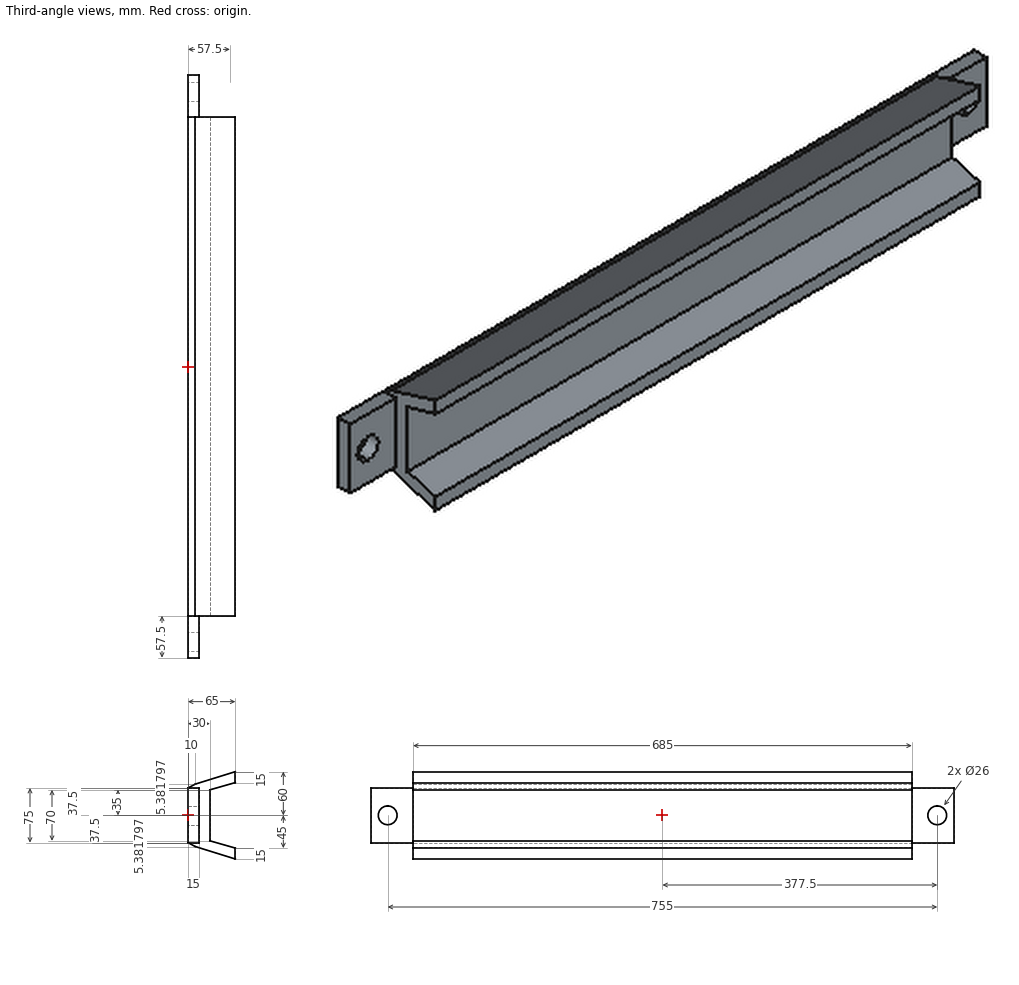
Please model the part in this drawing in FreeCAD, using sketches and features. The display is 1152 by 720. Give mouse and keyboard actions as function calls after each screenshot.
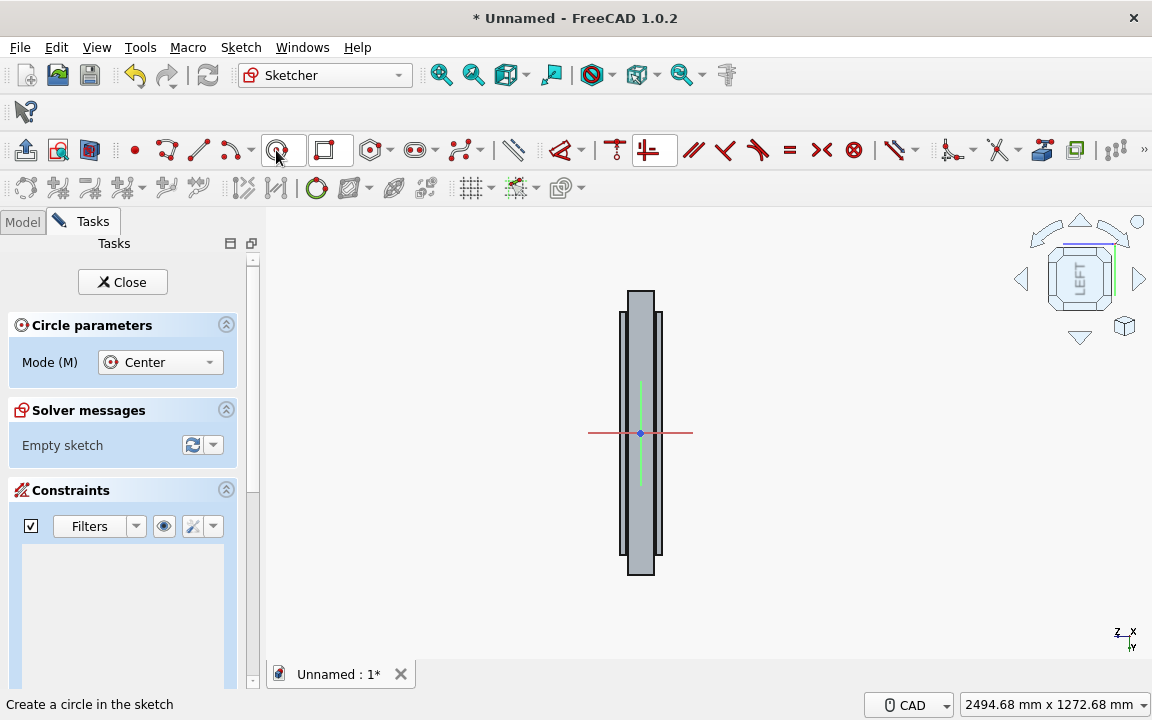
scroll(641, 567, up, 8)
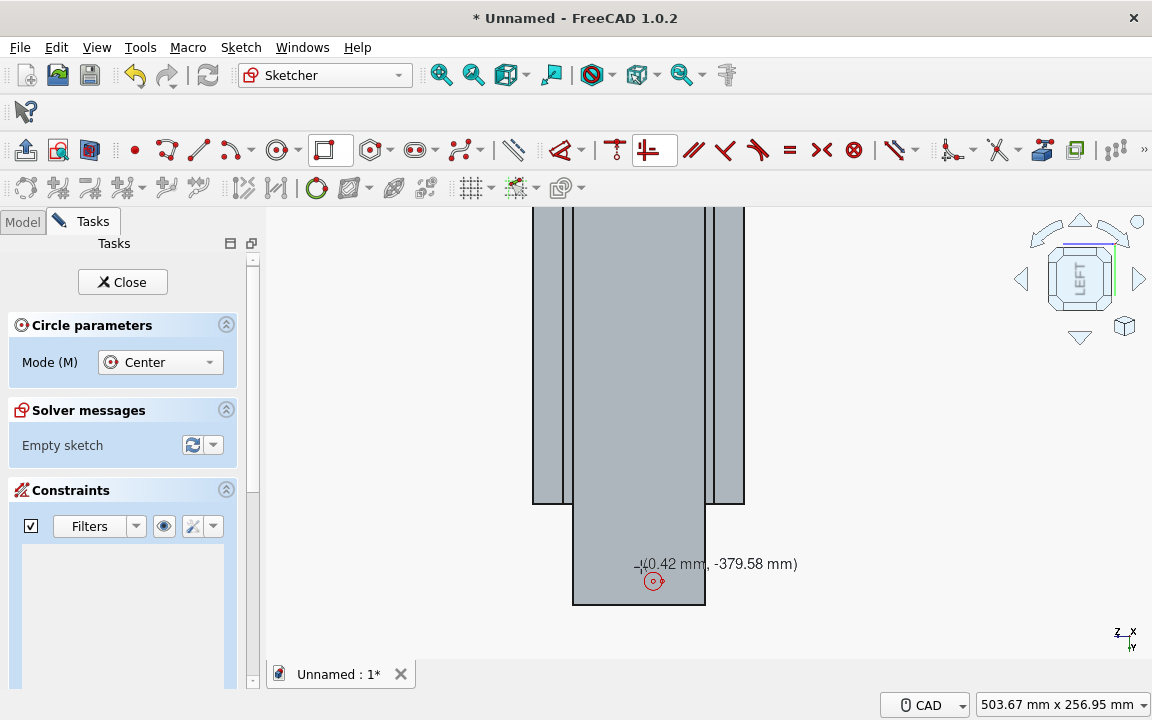
scroll(641, 568, down, 8)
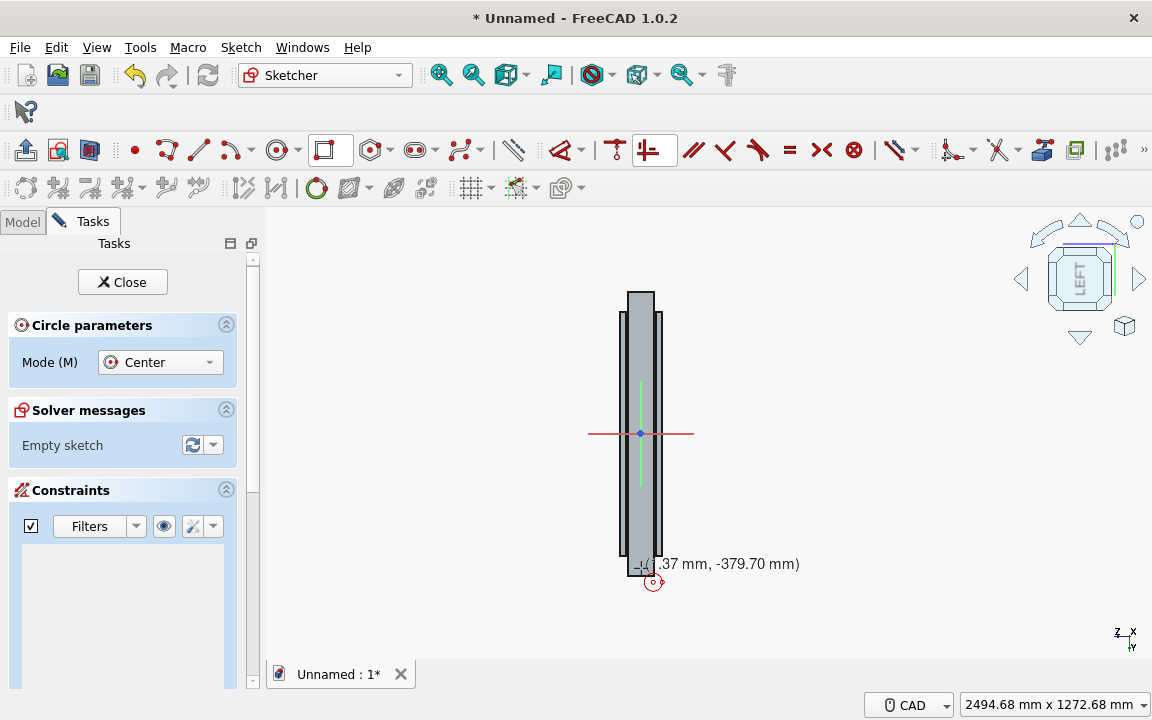
click(641, 568)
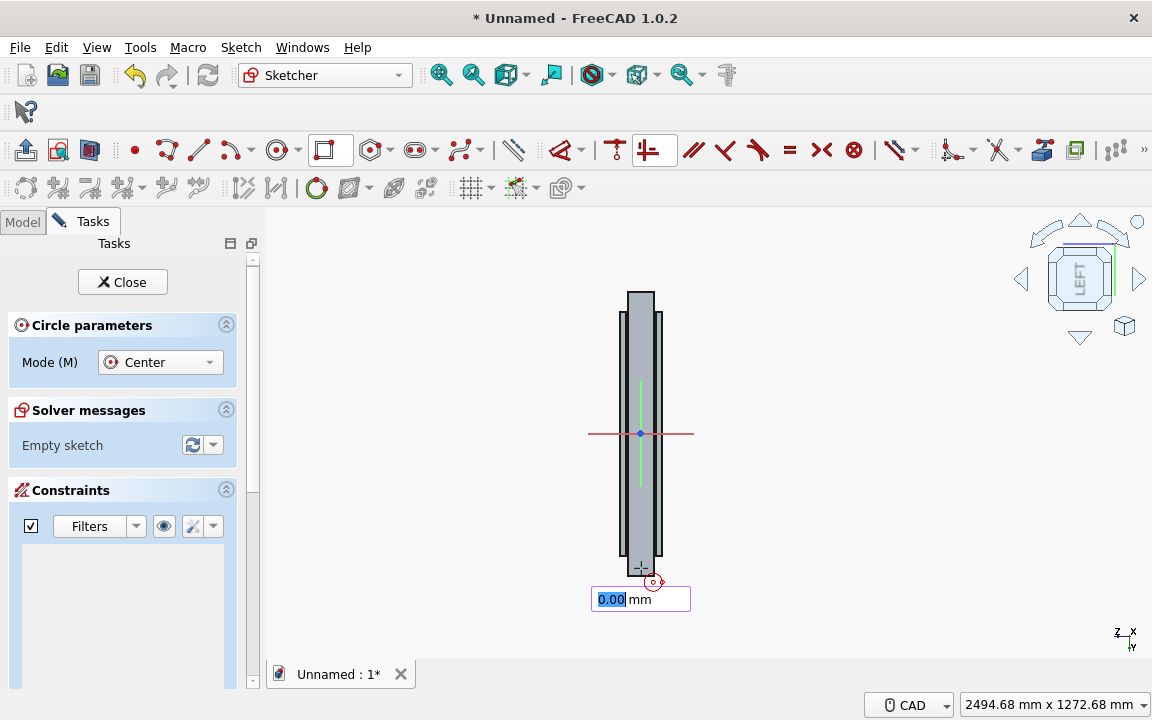
scroll(645, 566, up, 7)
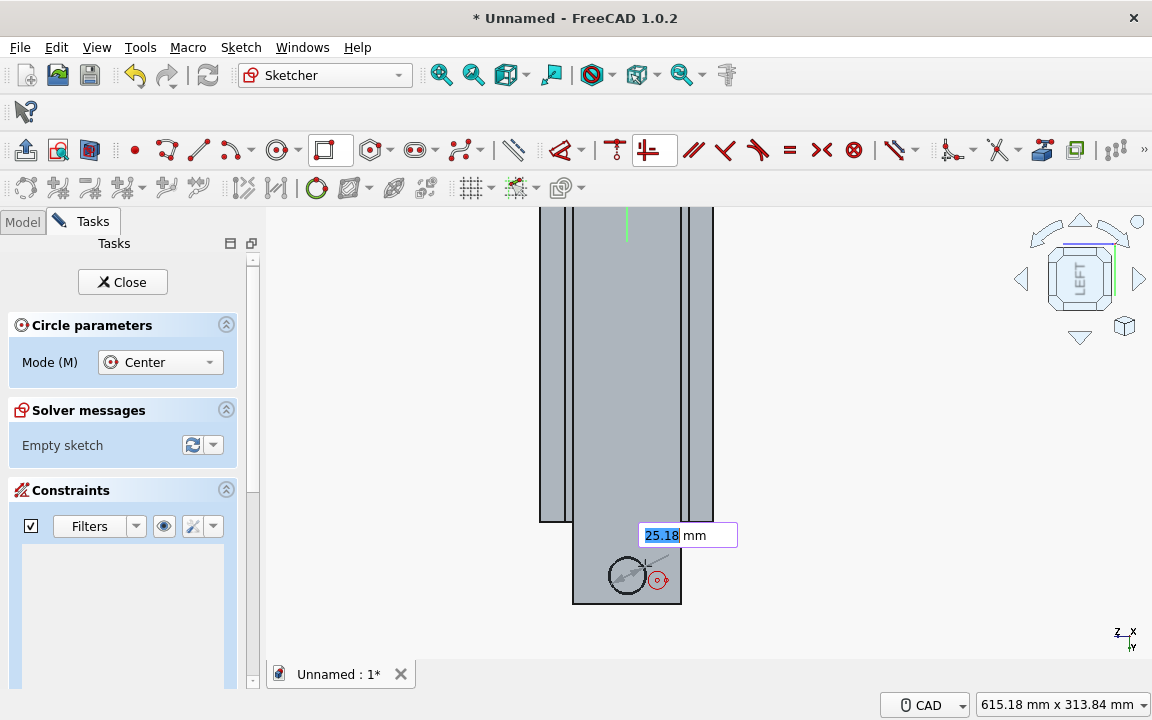
click(644, 566)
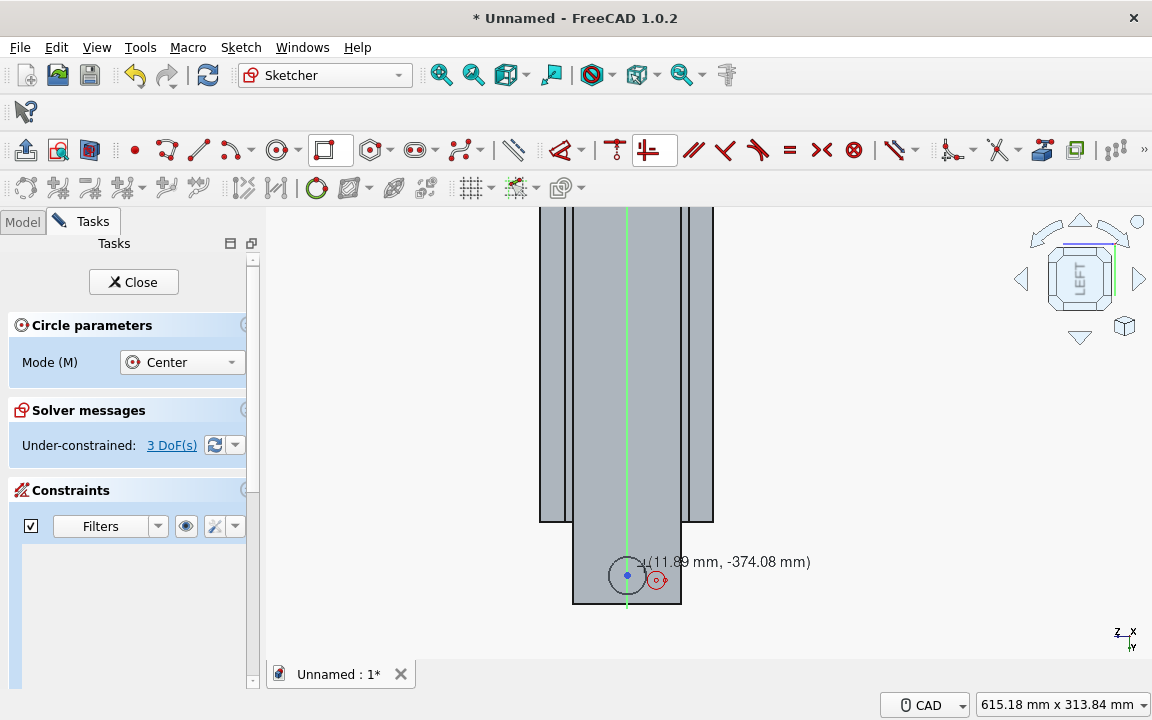
scroll(645, 565, down, 7)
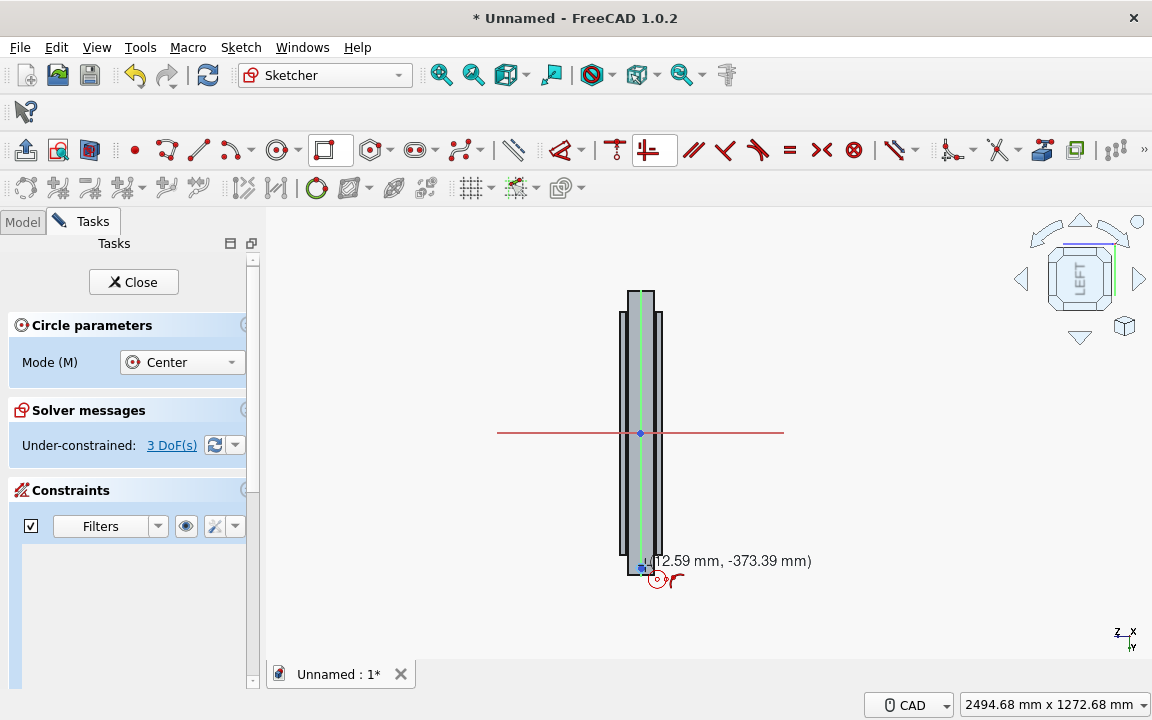
scroll(641, 299, up, 8)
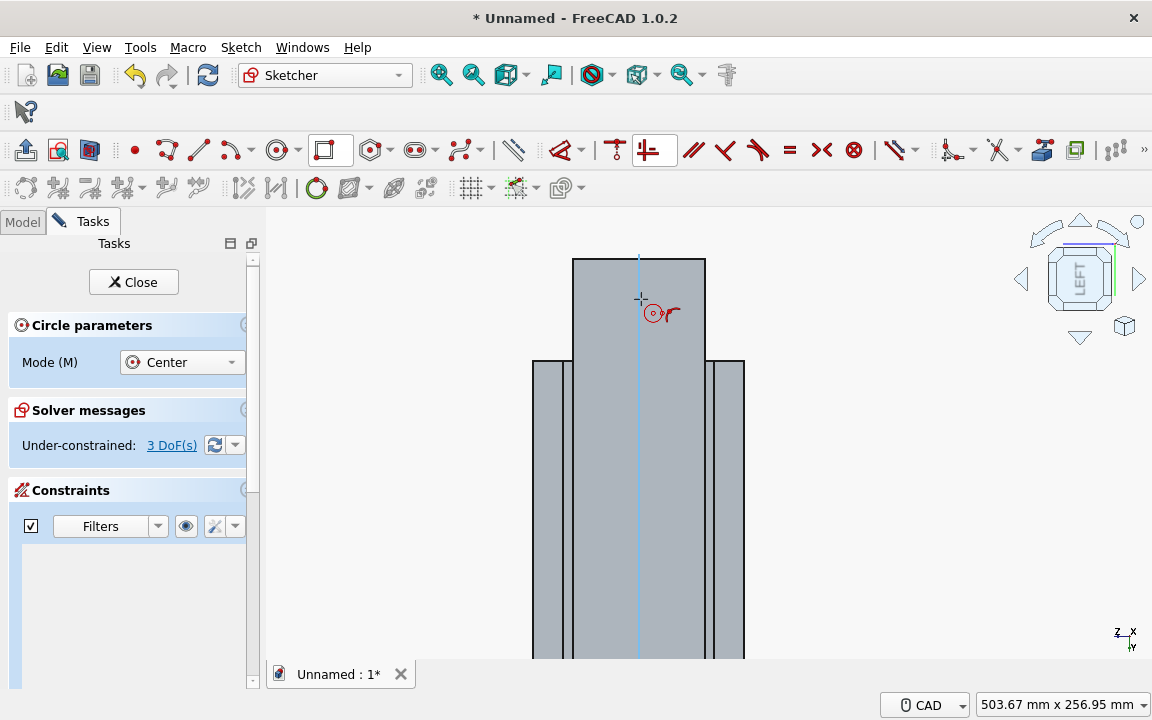
scroll(641, 299, down, 8)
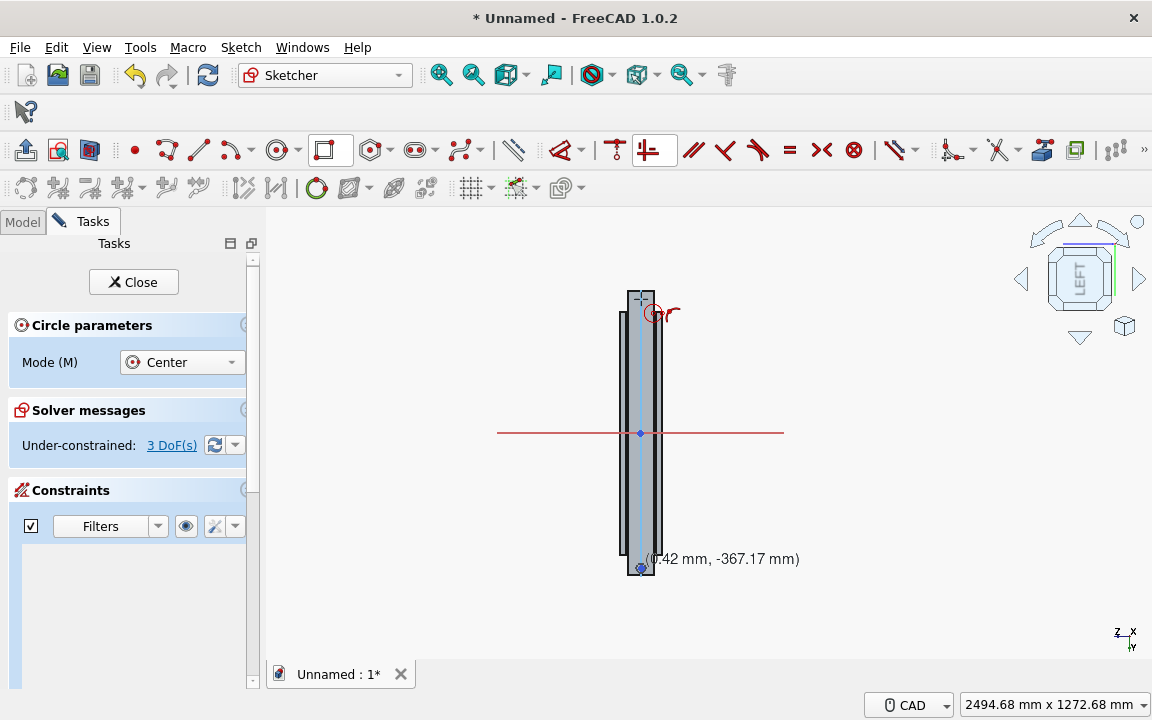
click(641, 299)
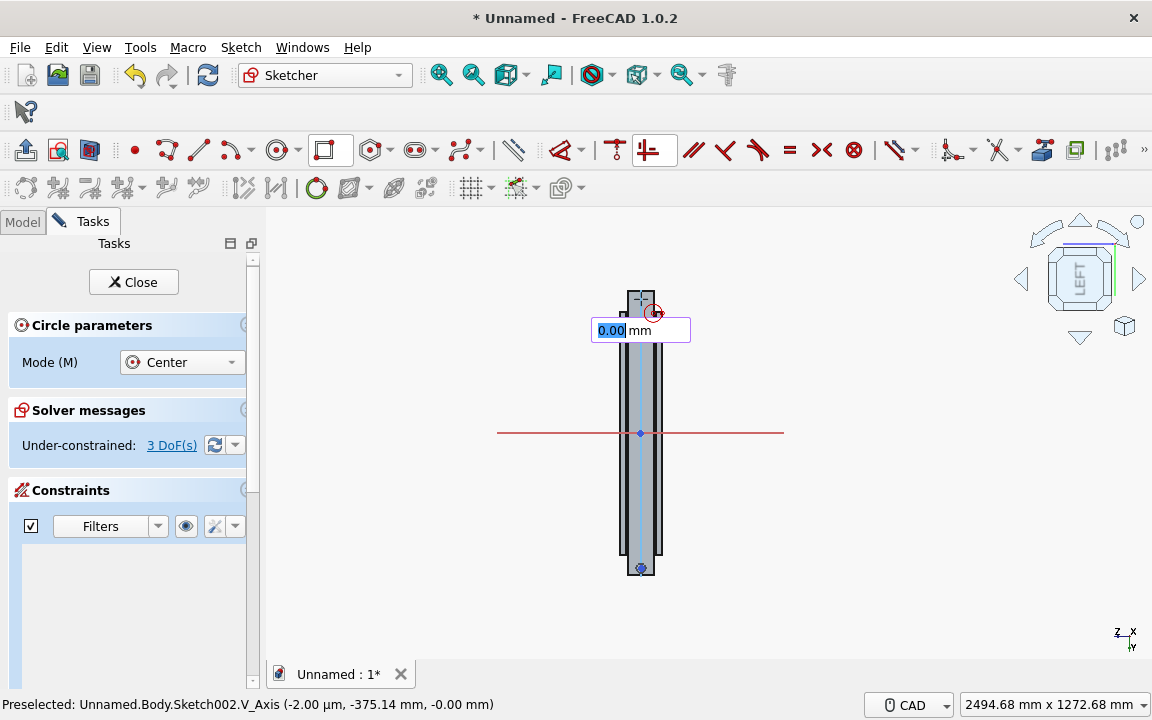
scroll(645, 298, up, 7)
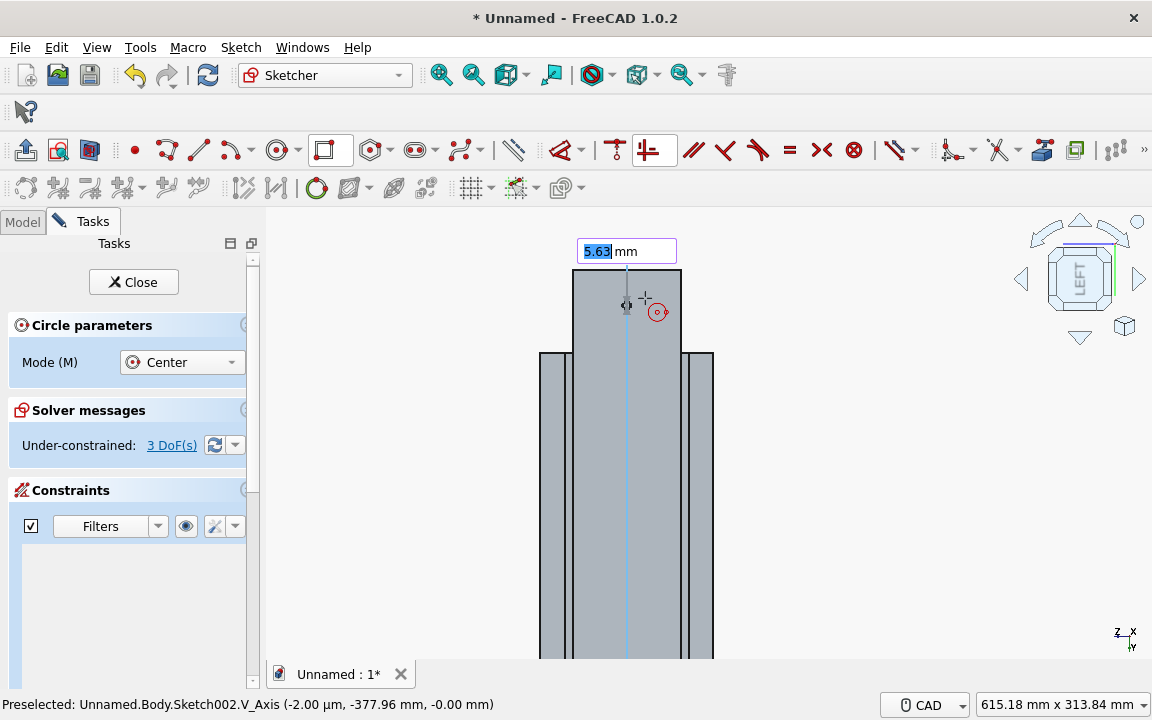
click(644, 296)
key(Escape)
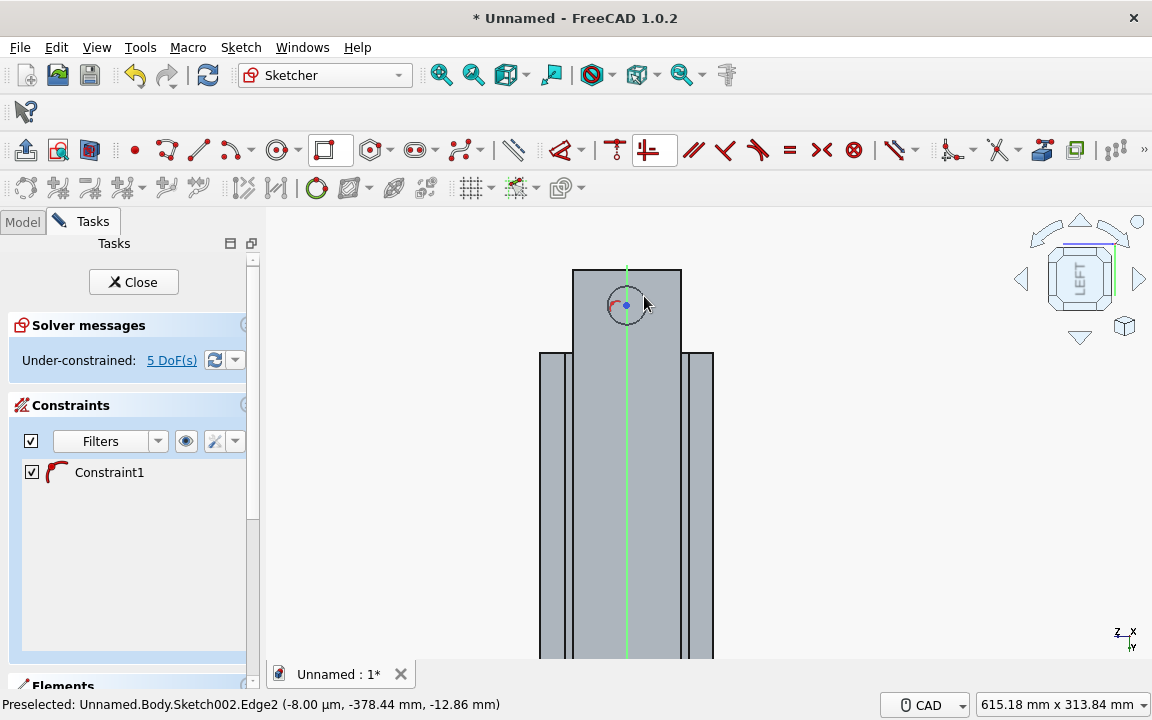
scroll(645, 298, down, 7)